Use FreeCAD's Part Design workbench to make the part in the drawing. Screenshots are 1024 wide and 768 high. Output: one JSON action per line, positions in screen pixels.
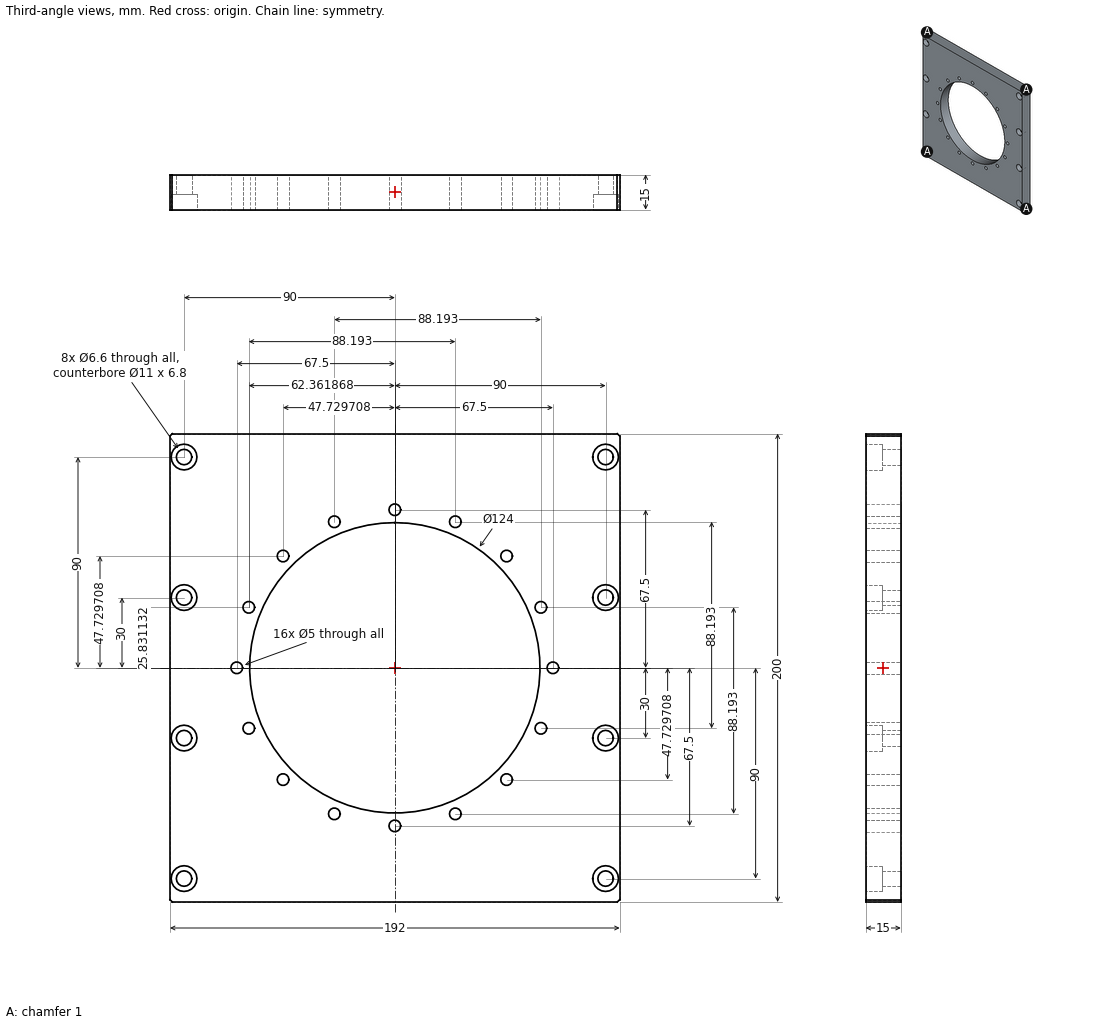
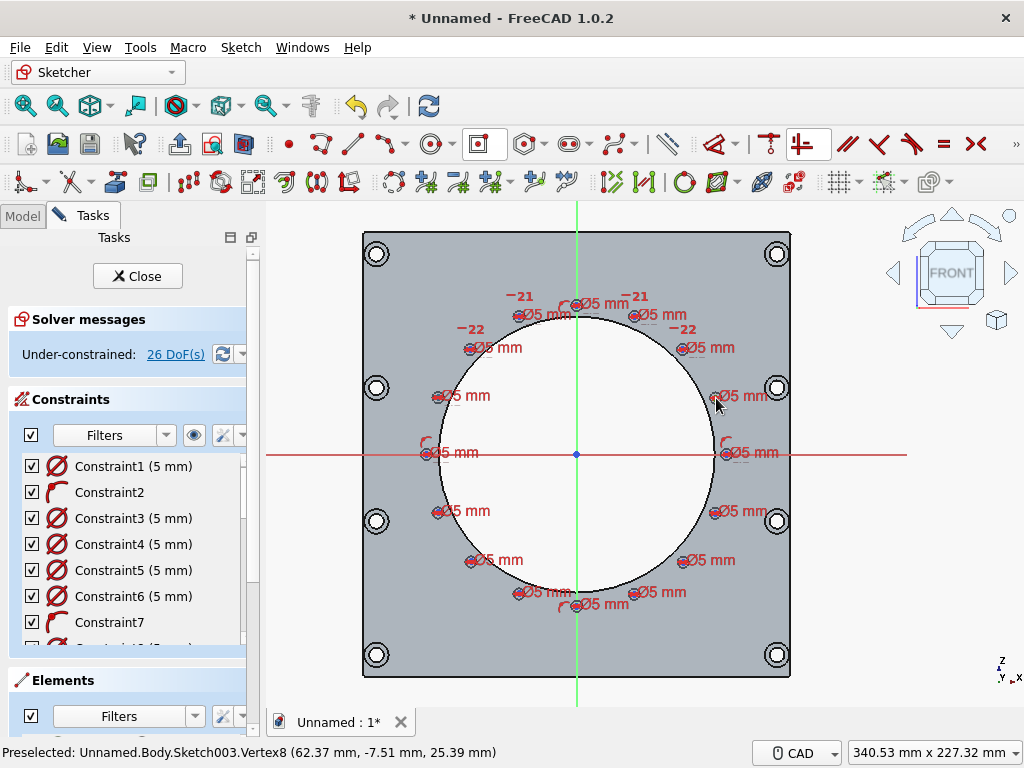
{"action": "left_click", "coordinate": [826, 144]}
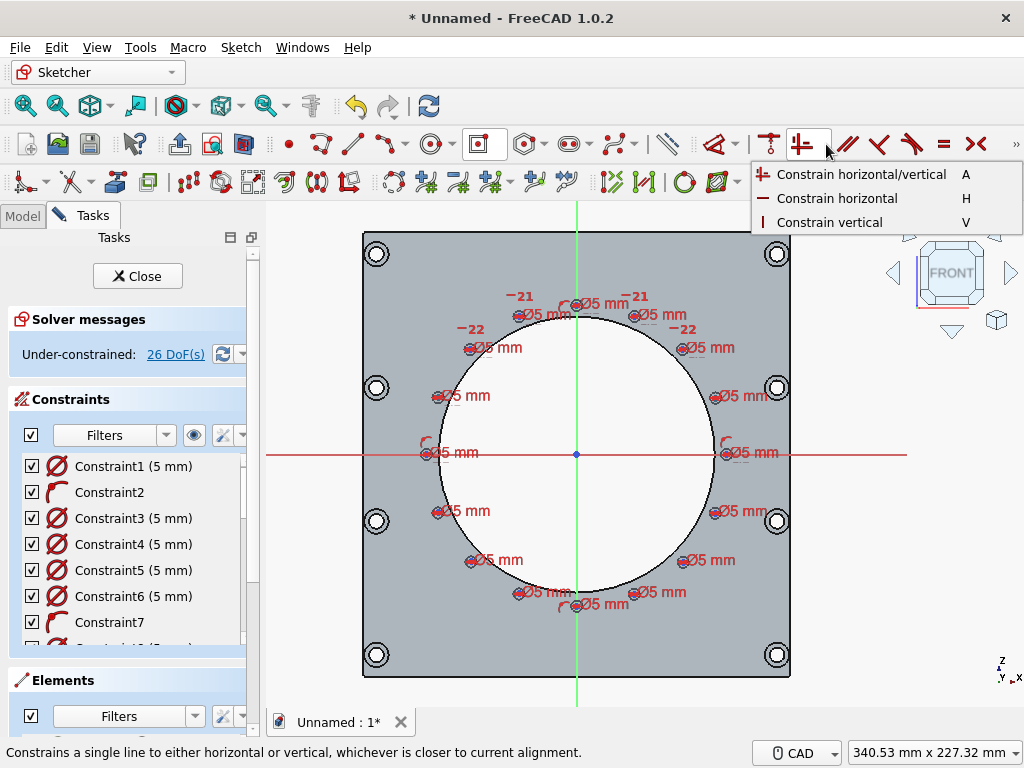
{"action": "left_click", "coordinate": [887, 198]}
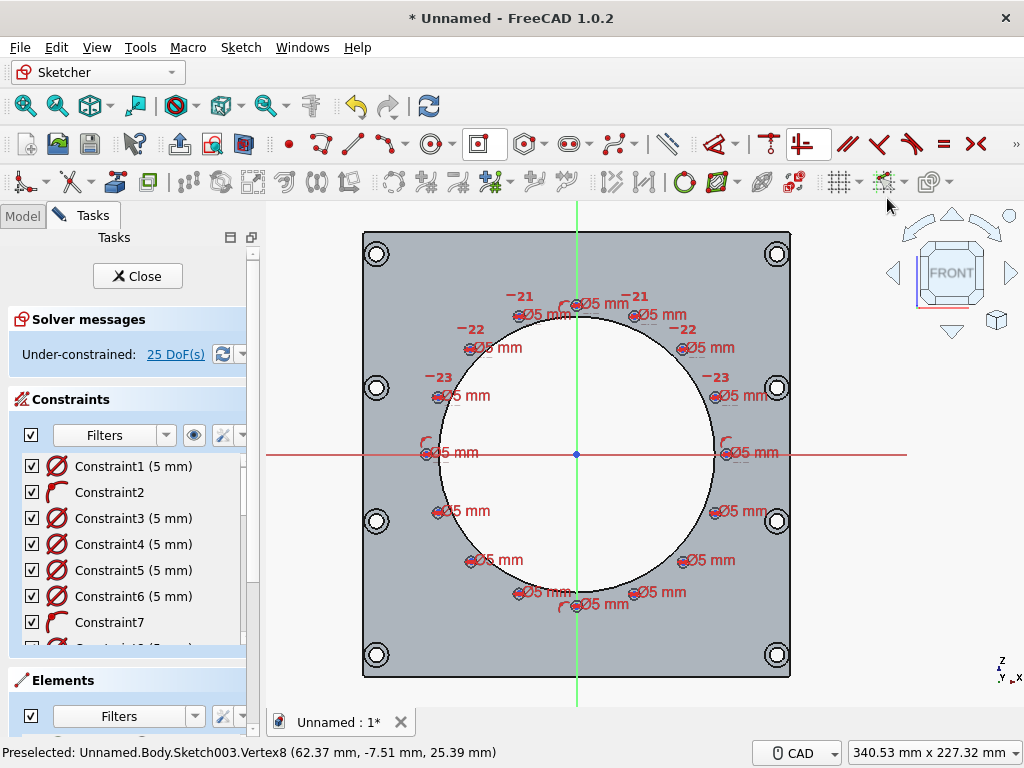
{"action": "left_click", "coordinate": [716, 398]}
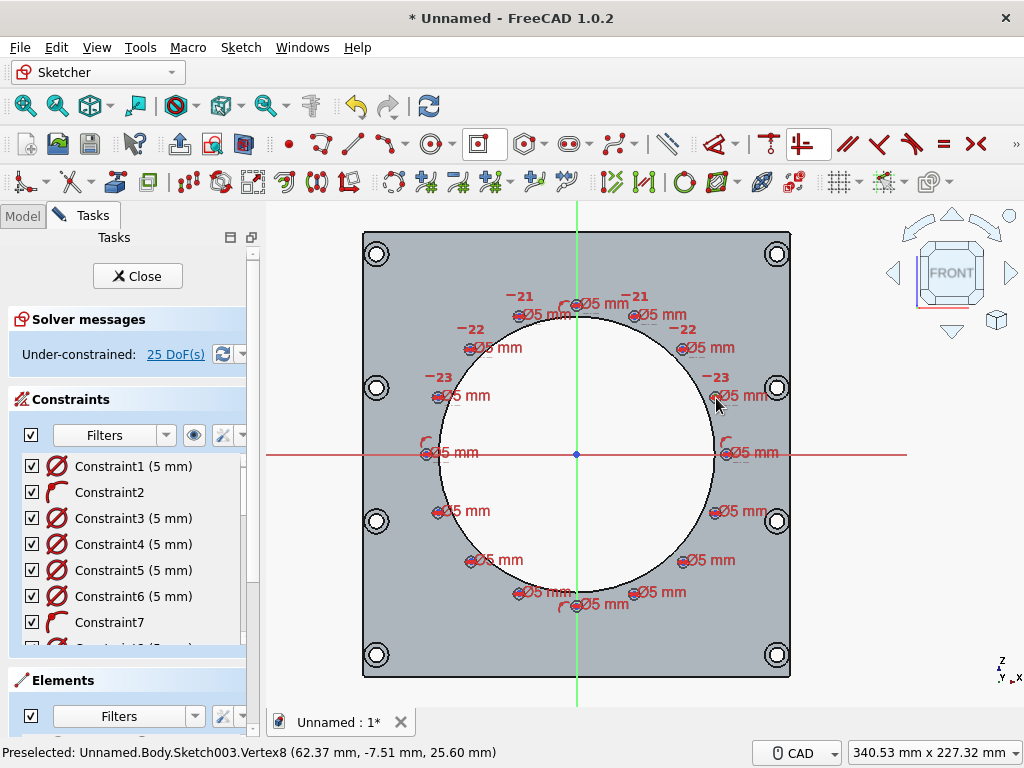
{"action": "left_click", "coordinate": [715, 513]}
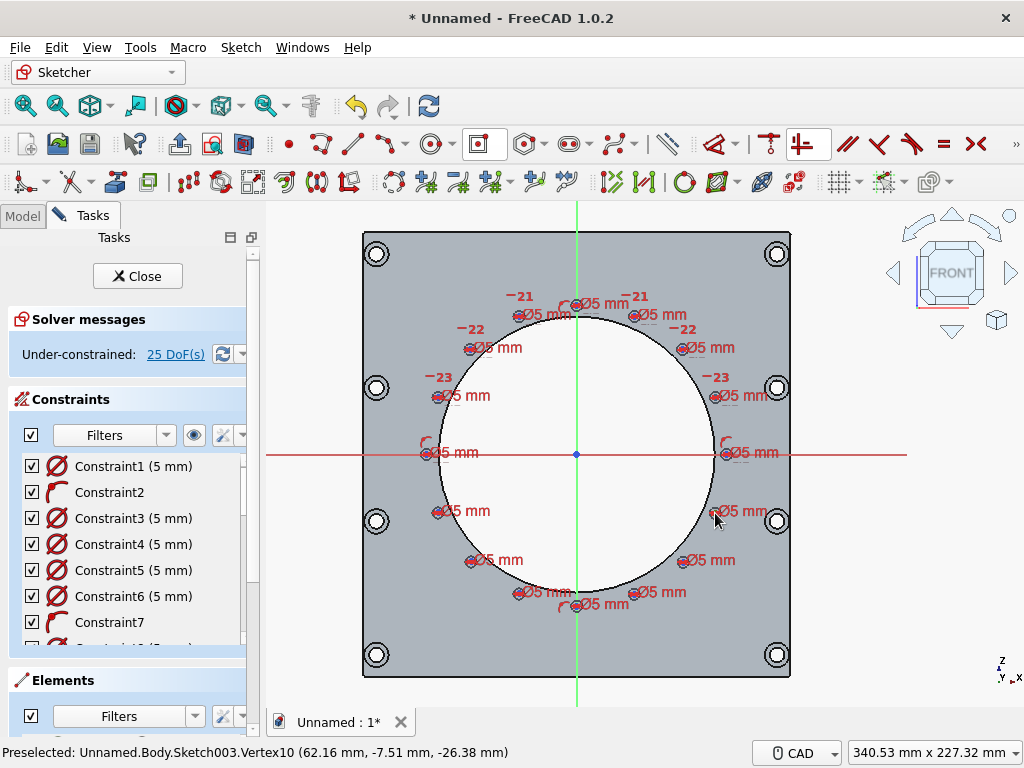
{"action": "left_click", "coordinate": [826, 144]}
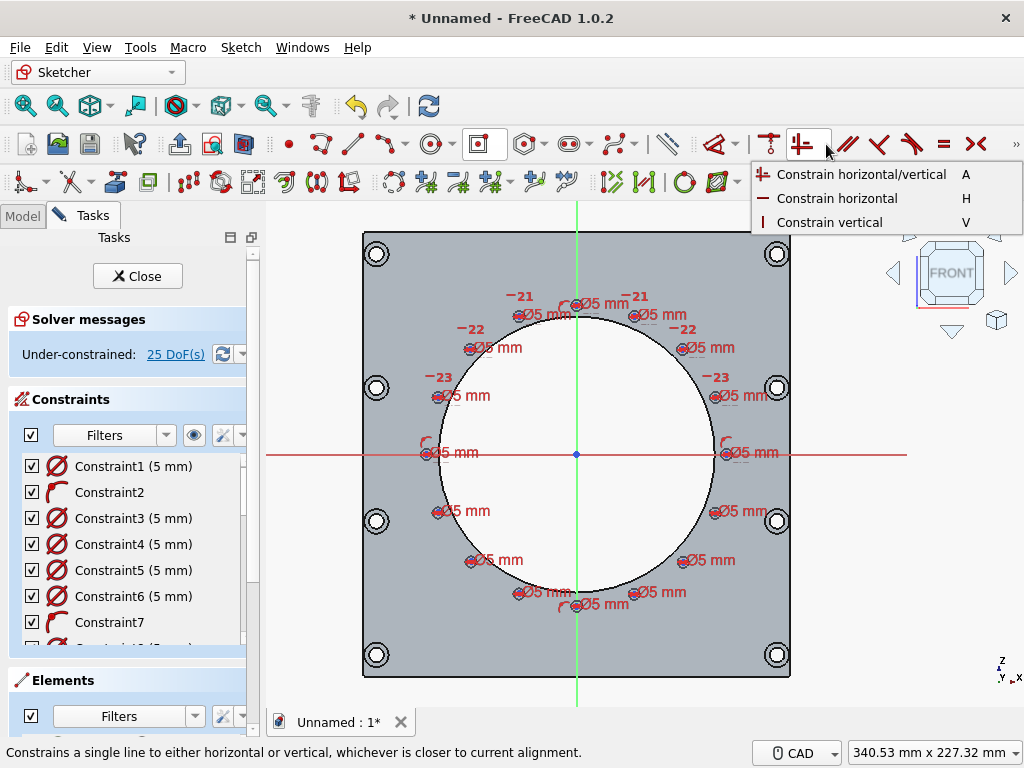
{"action": "left_click", "coordinate": [887, 222]}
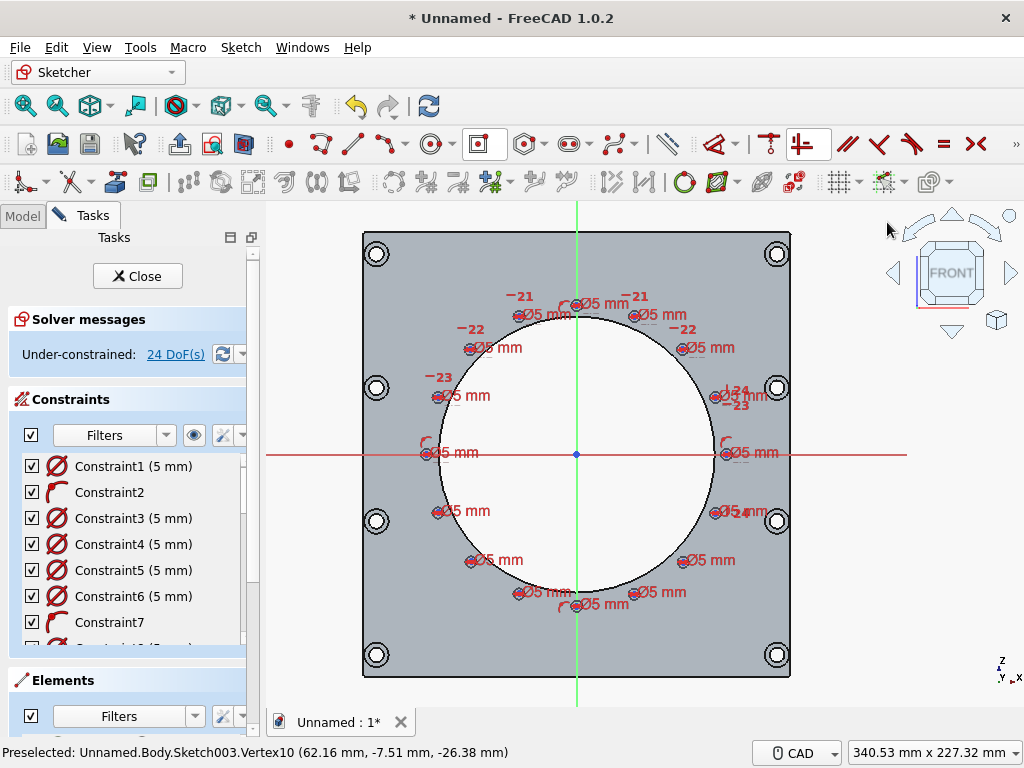
{"action": "left_click", "coordinate": [683, 350]}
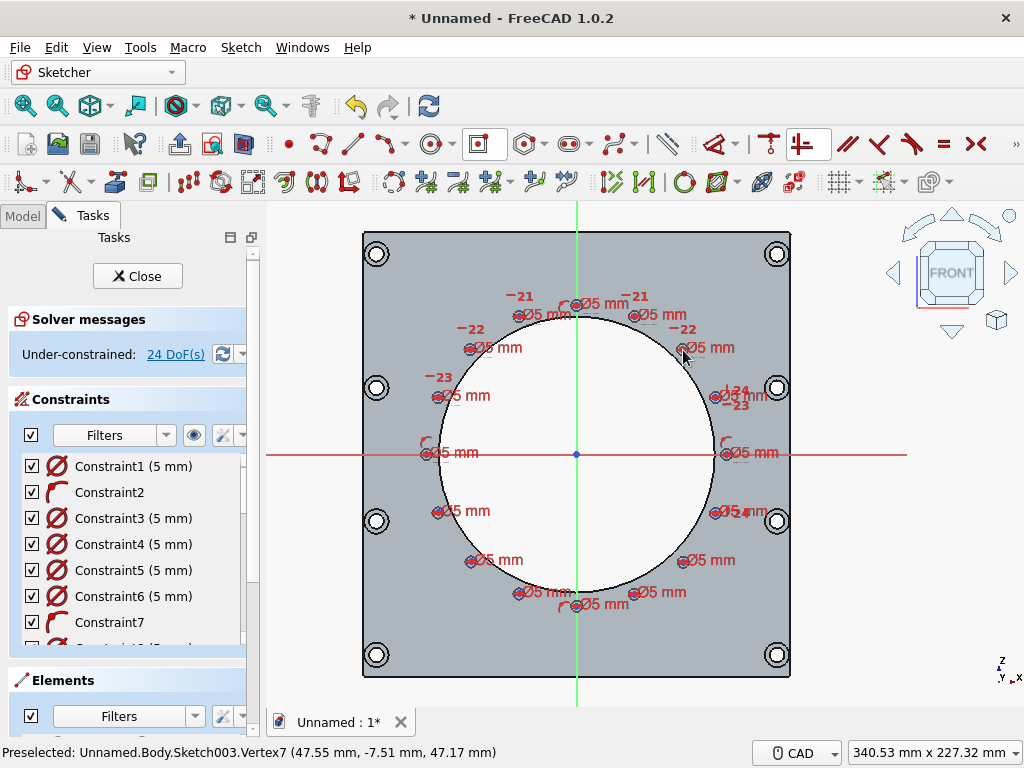
{"action": "left_click", "coordinate": [683, 562]}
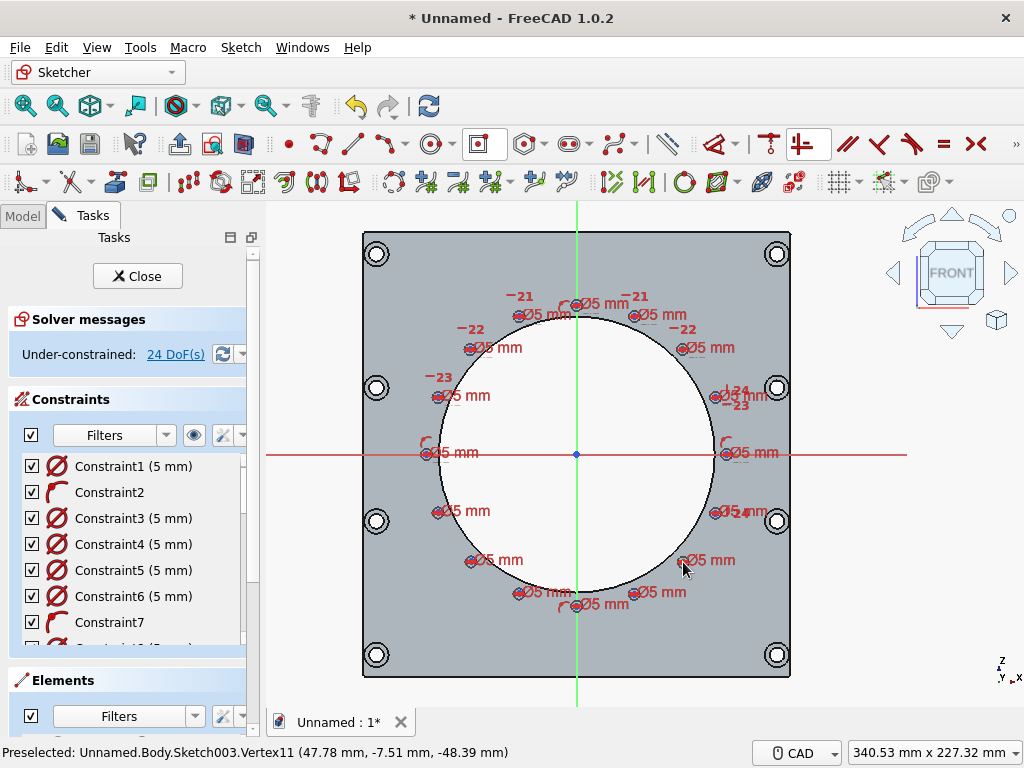
{"action": "left_click", "coordinate": [826, 144]}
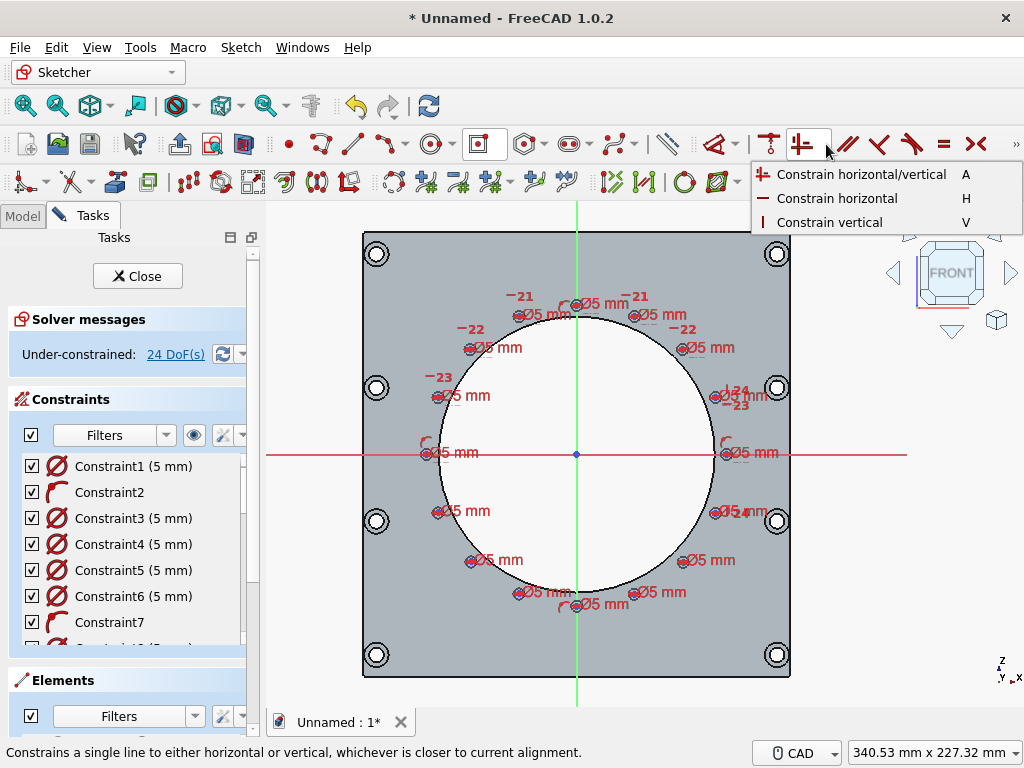
{"action": "left_click", "coordinate": [887, 222]}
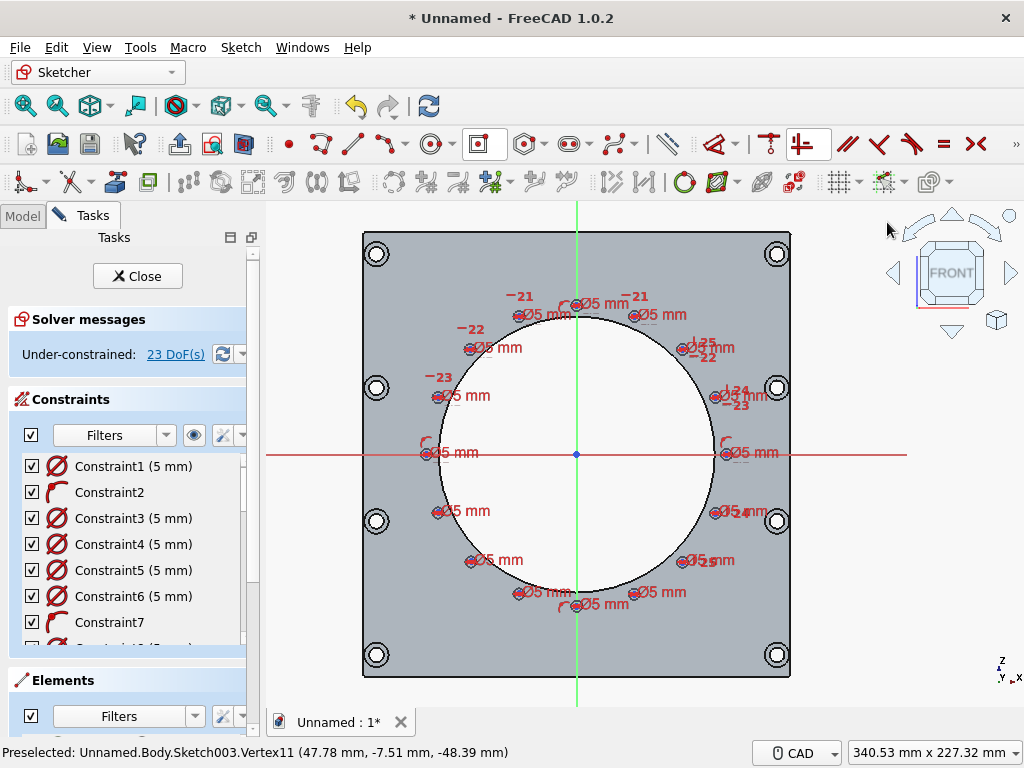
{"action": "left_click", "coordinate": [634, 594]}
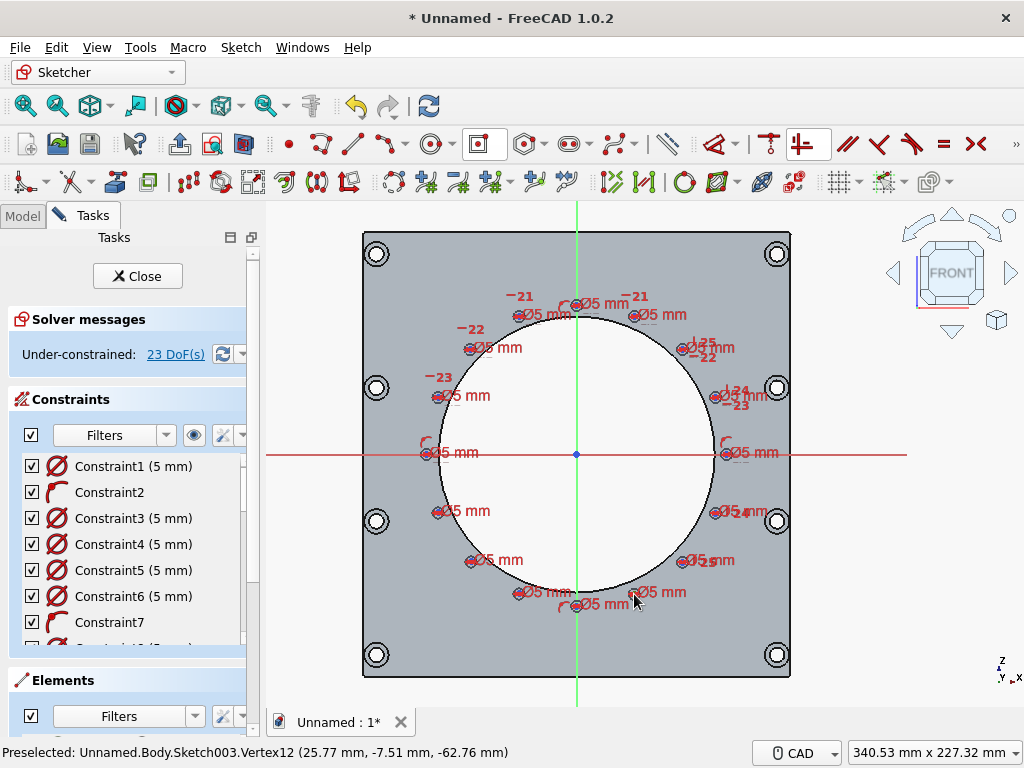
{"action": "left_click", "coordinate": [519, 594]}